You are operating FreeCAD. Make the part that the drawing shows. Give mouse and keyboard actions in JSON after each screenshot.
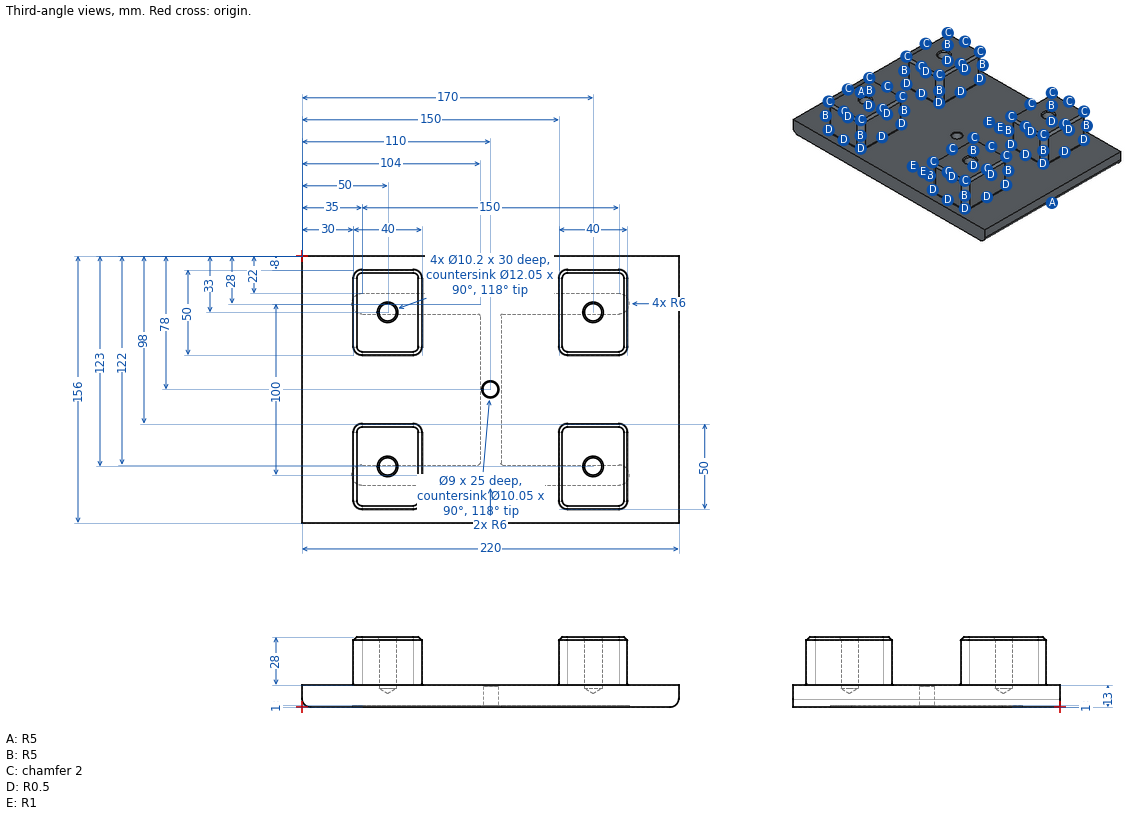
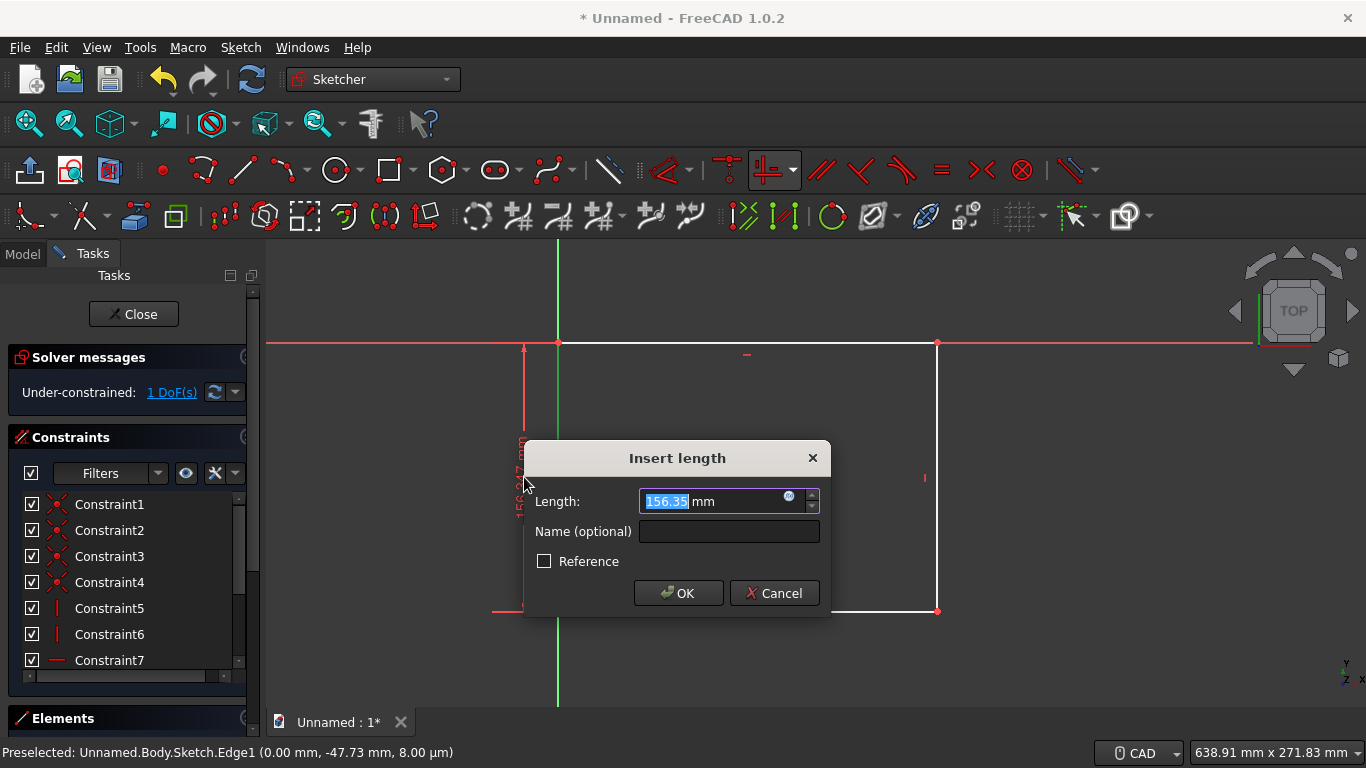
{"action": "type", "text": "156"}
{"action": "key", "text": "Return"}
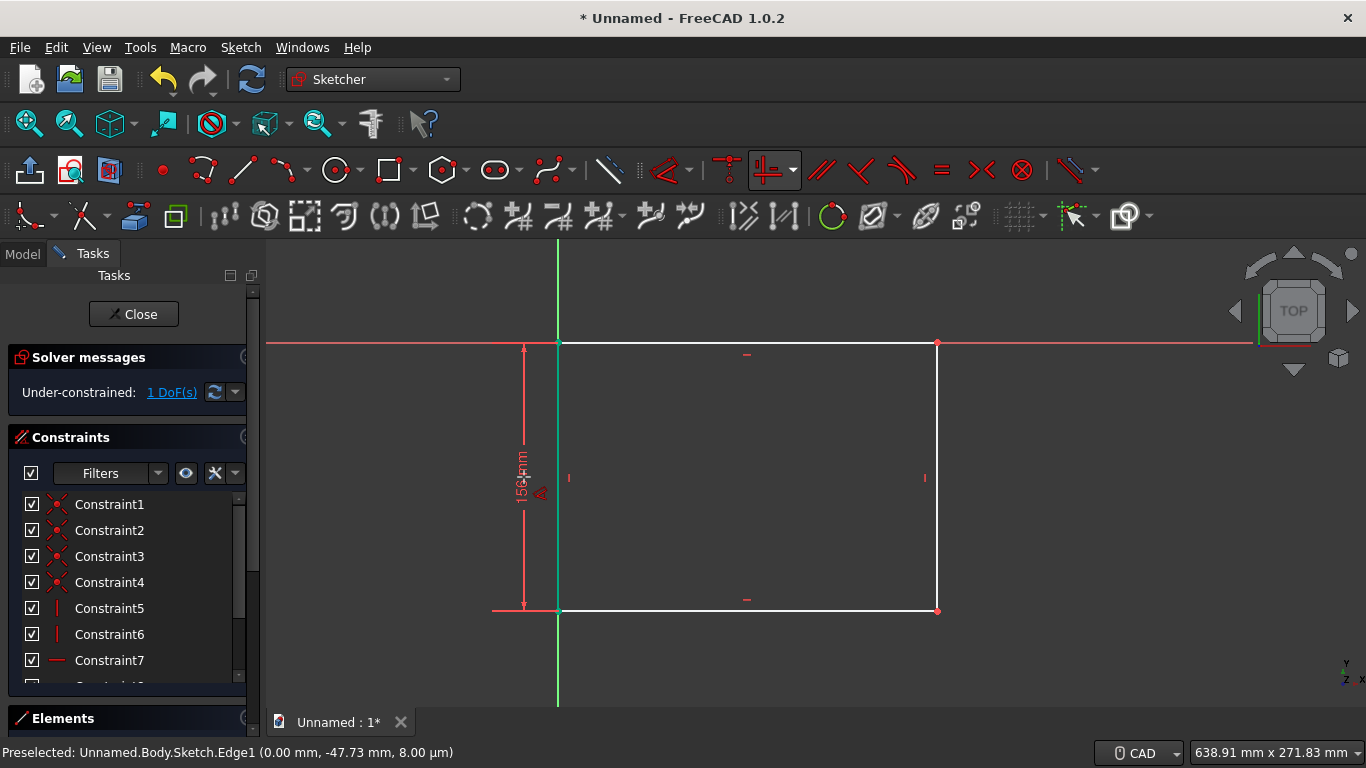
{"action": "left_click", "coordinate": [672, 611]}
{"action": "left_click", "coordinate": [748, 645]}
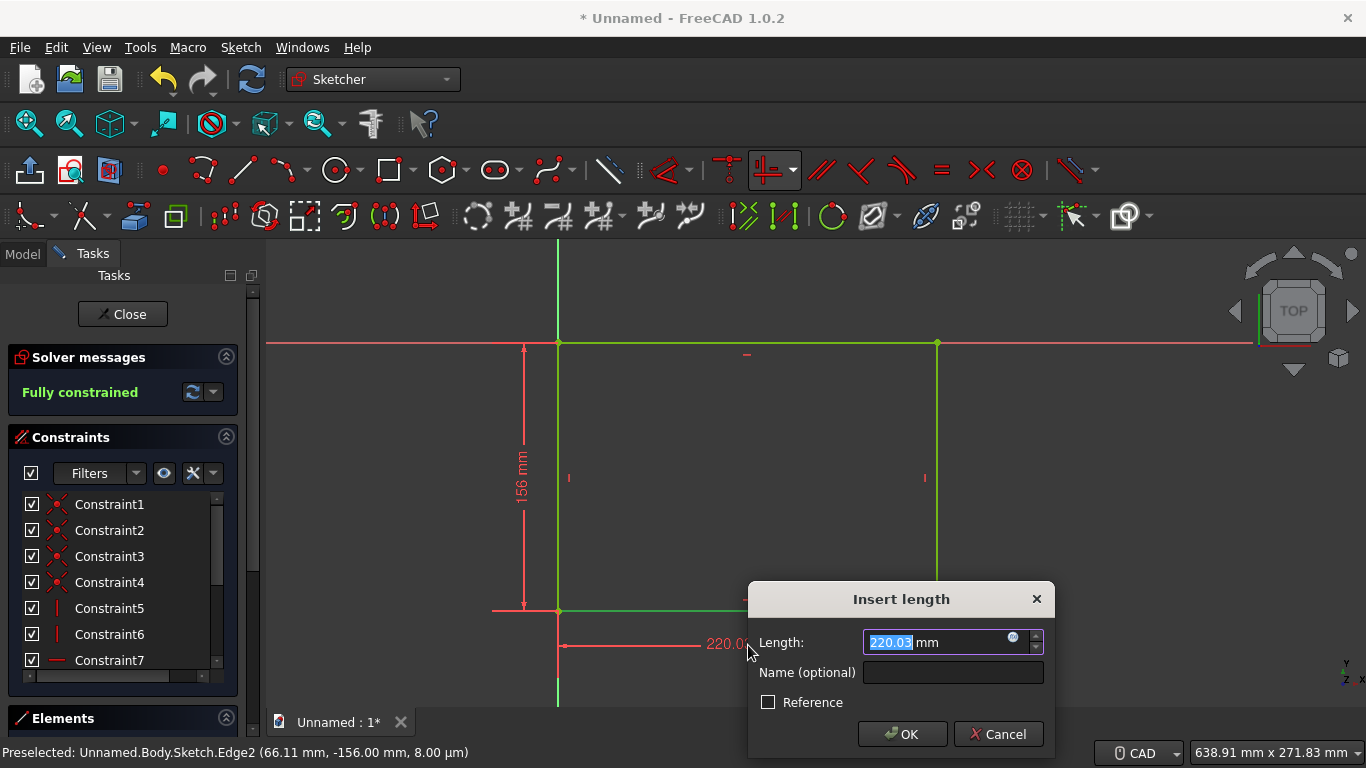
{"action": "type", "text": "220"}
{"action": "key", "text": "Return"}
{"action": "key", "text": "Escape"}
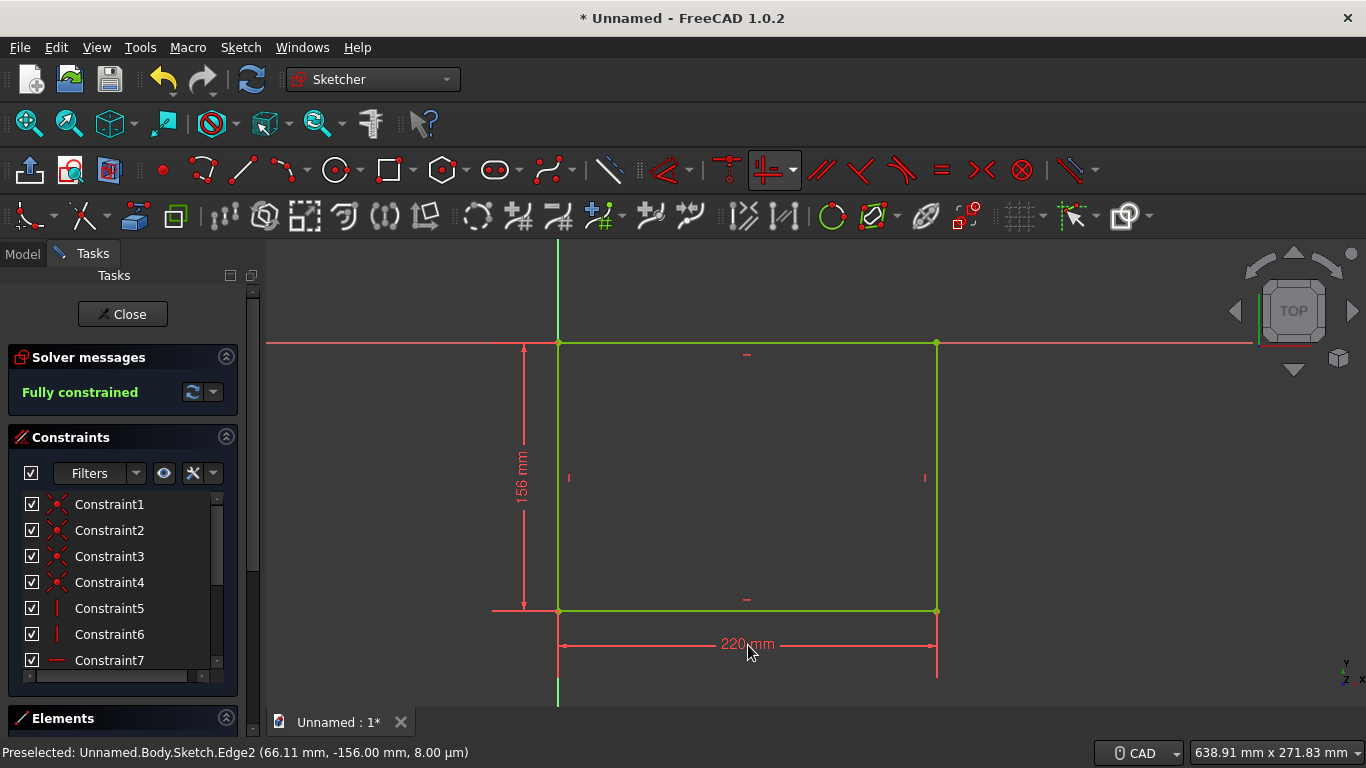
{"action": "left_click", "coordinate": [123, 314]}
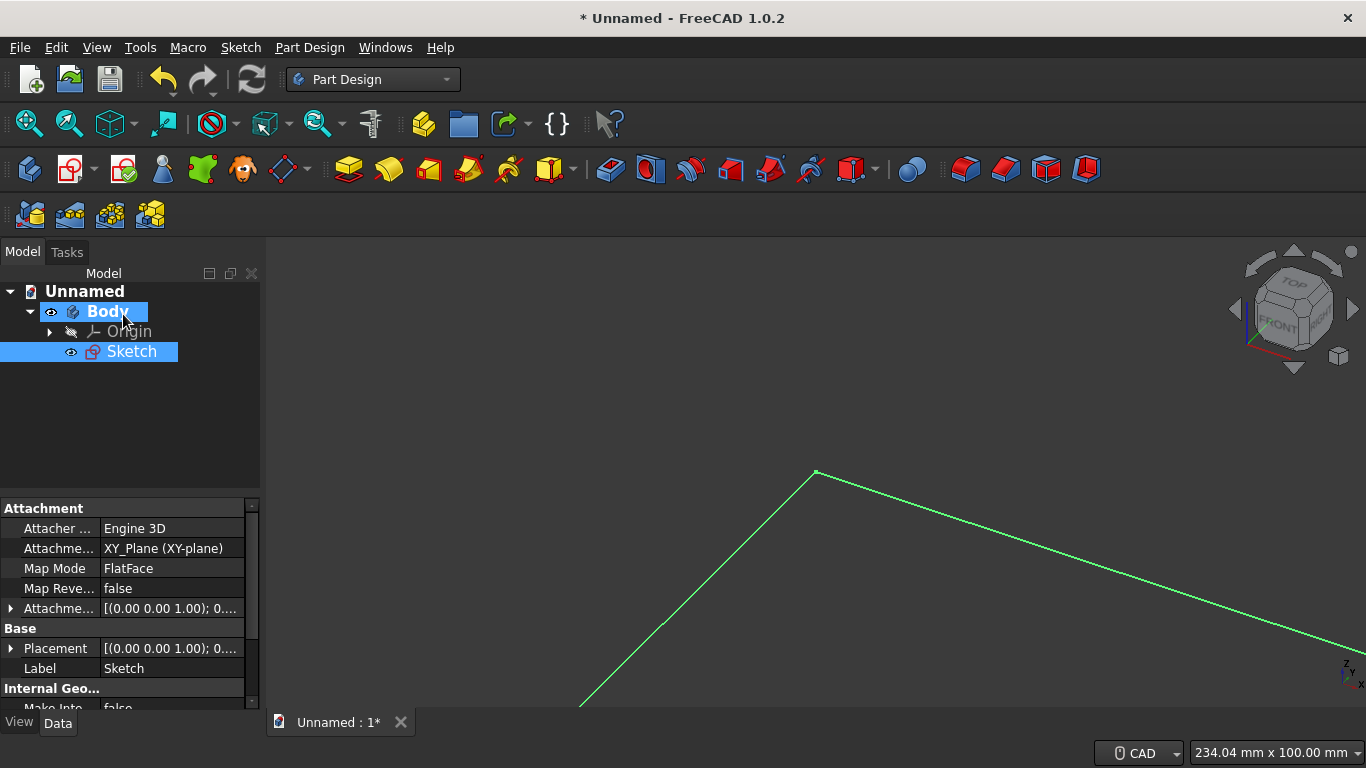
{"action": "left_click", "coordinate": [350, 170]}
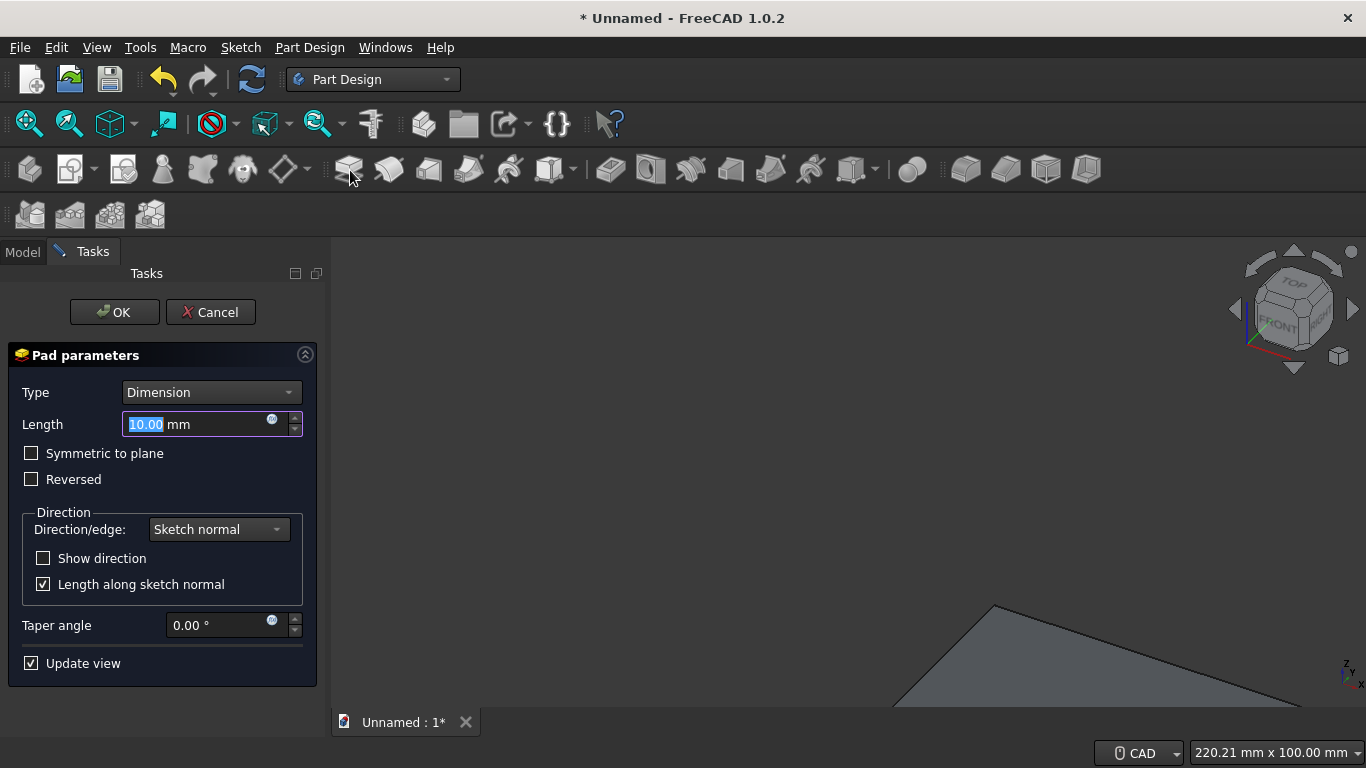
{"action": "type", "text": "13"}
{"action": "key", "text": "Tab"}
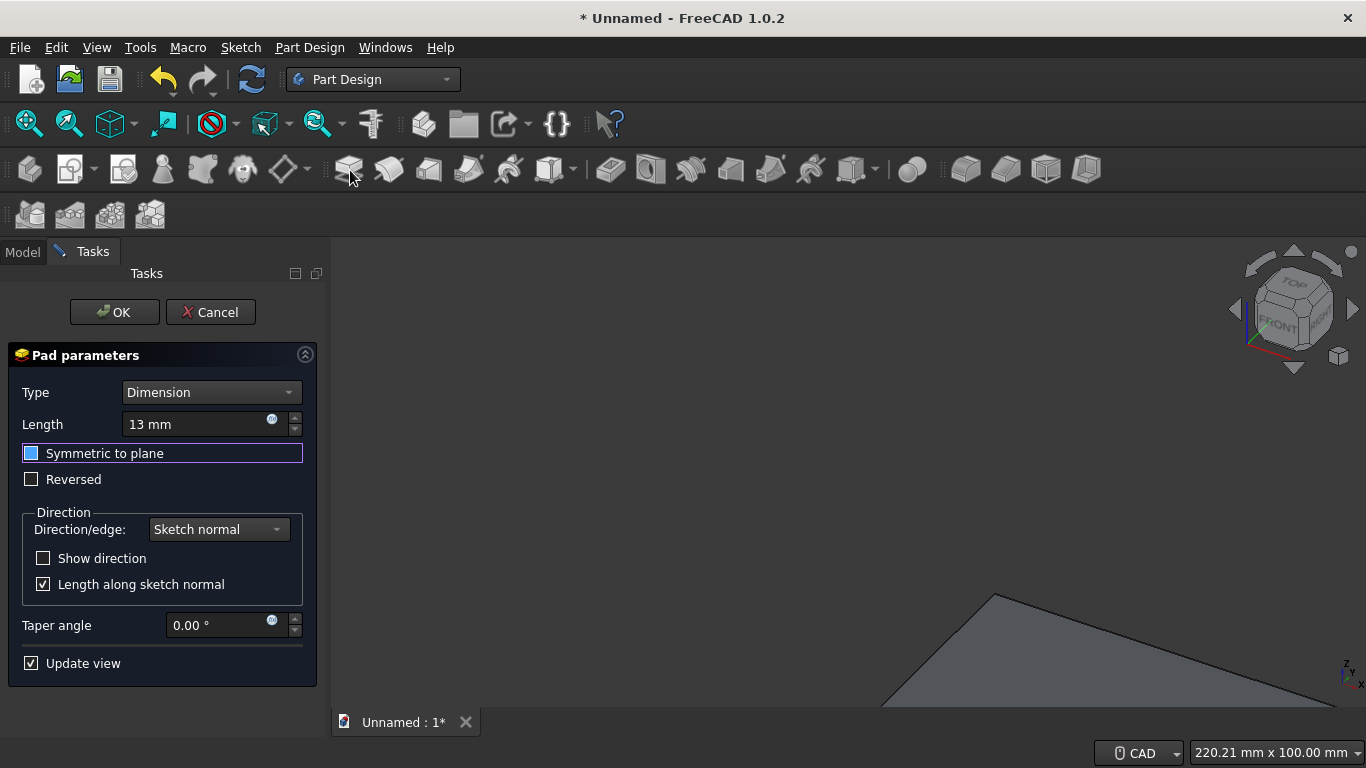
{"action": "left_click", "coordinate": [115, 312]}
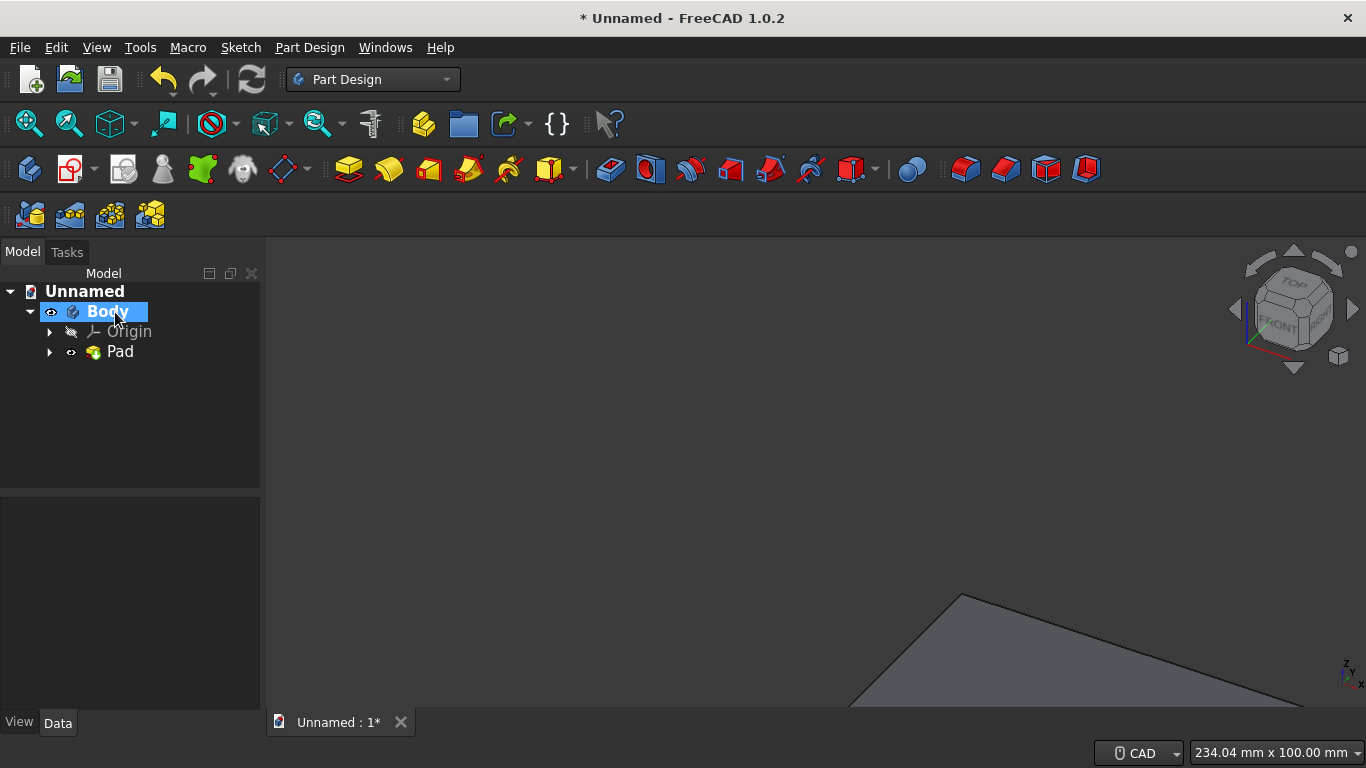
{"action": "left_click", "coordinate": [30, 124]}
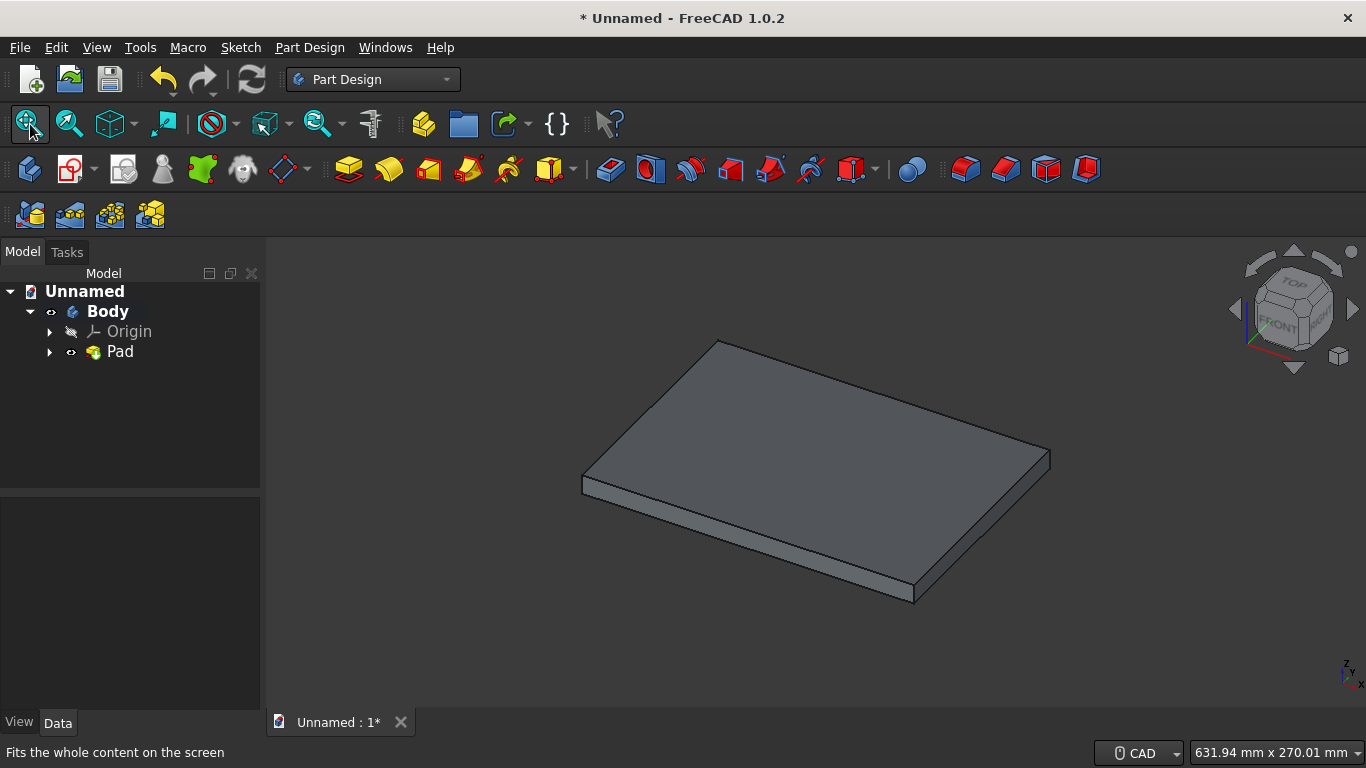
{"action": "left_click", "coordinate": [863, 477]}